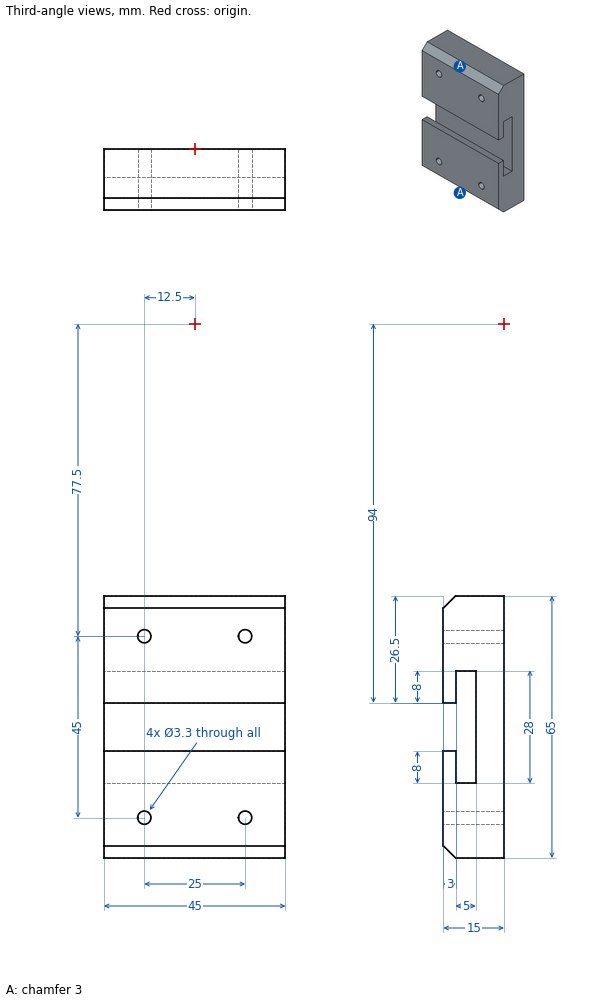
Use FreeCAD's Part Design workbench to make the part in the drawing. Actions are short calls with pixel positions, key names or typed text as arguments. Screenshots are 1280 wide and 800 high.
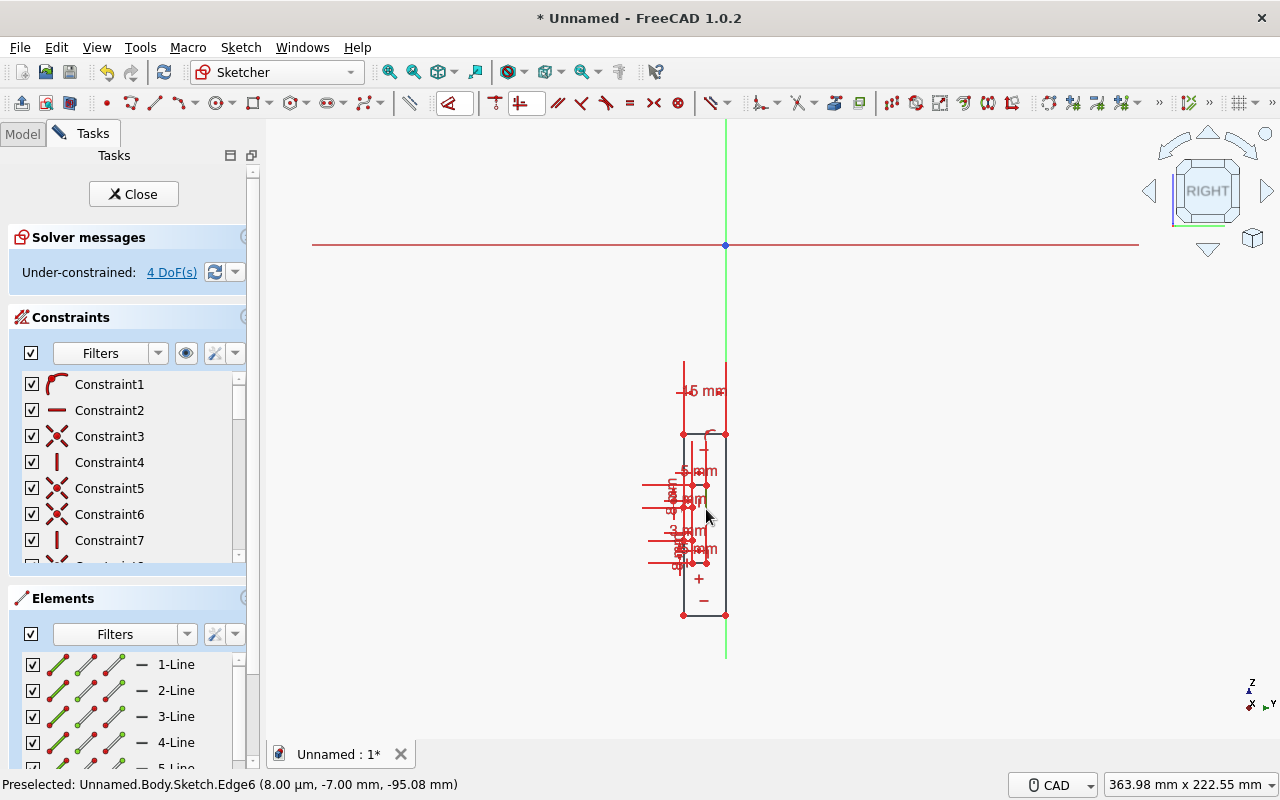
click(468, 104)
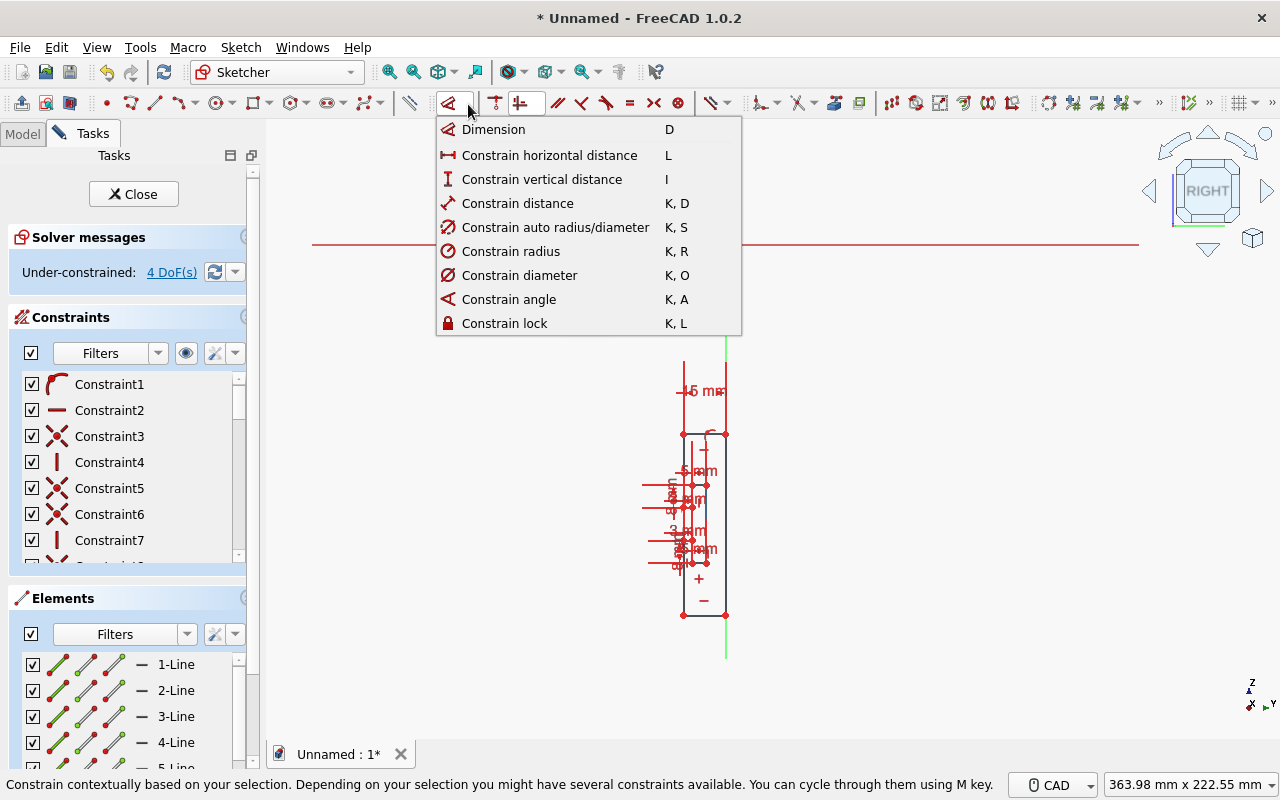
click(589, 179)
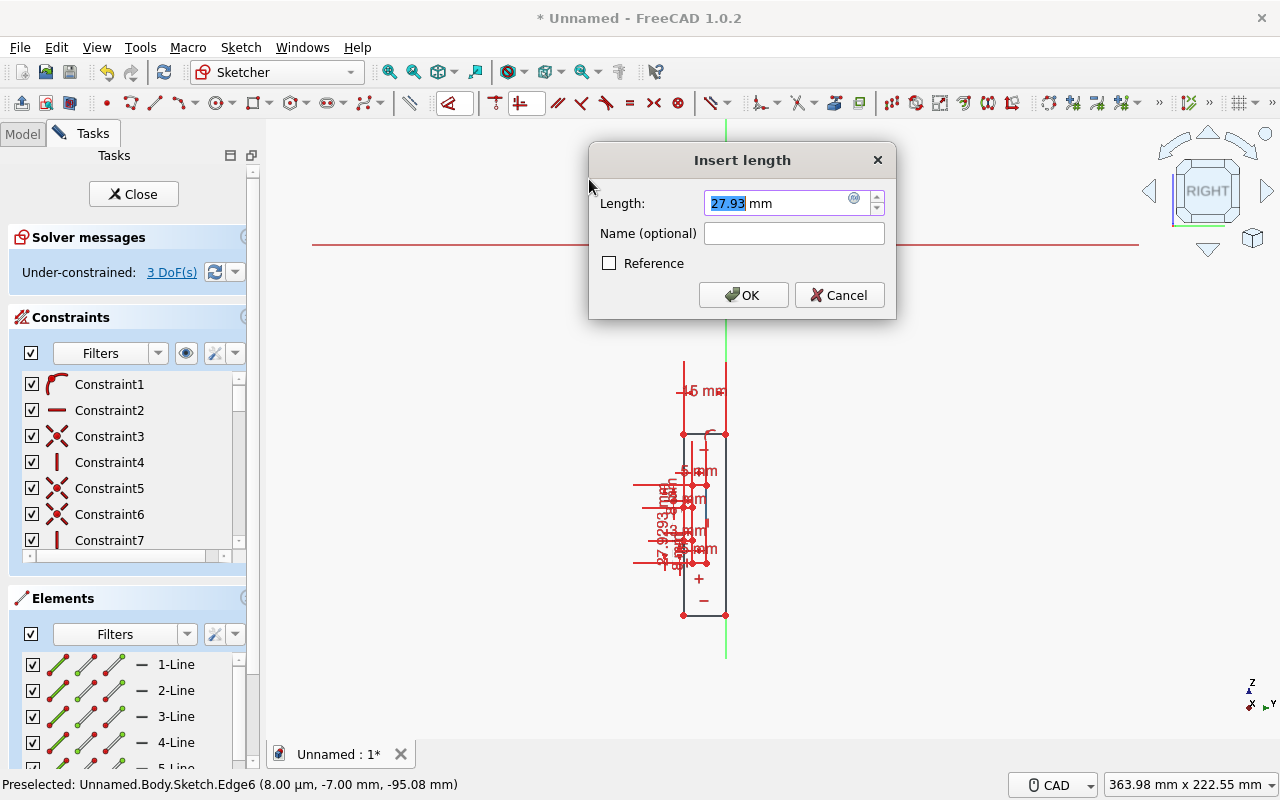
text(28)
key(Return)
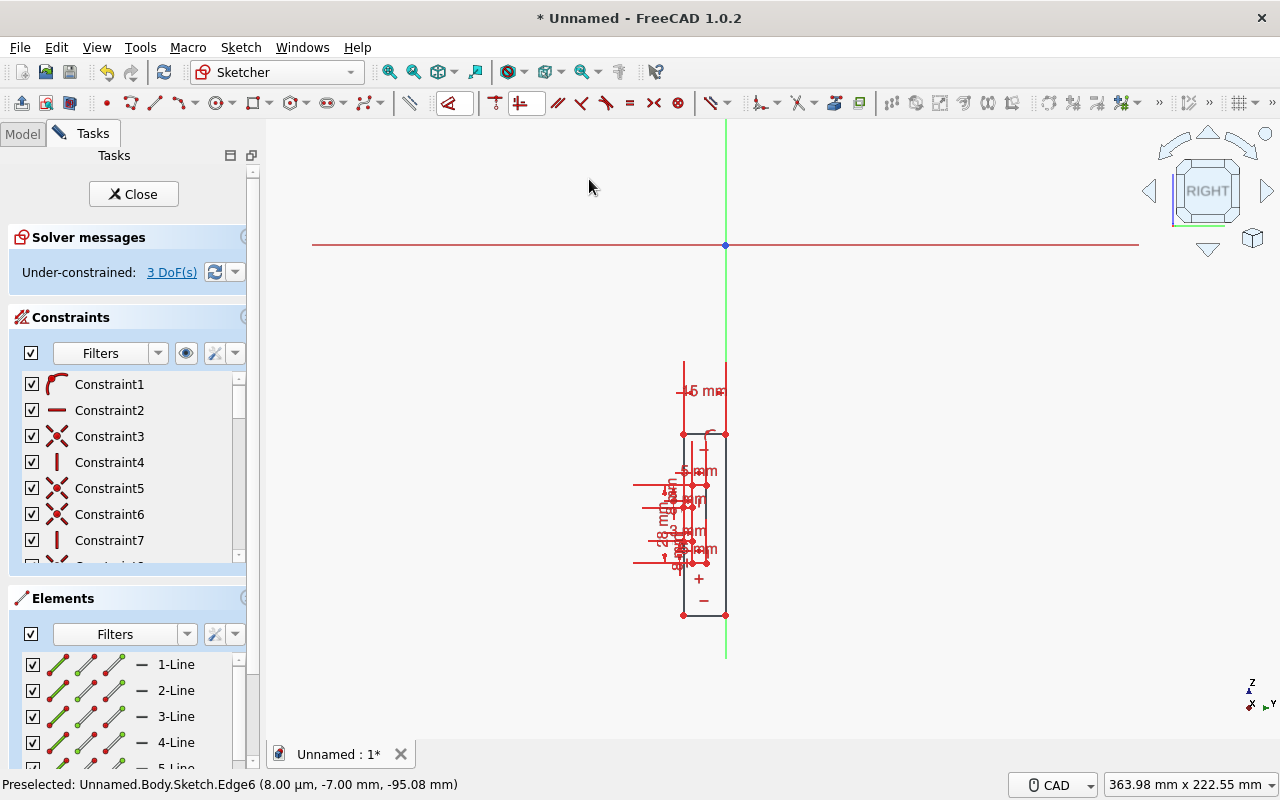
click(726, 561)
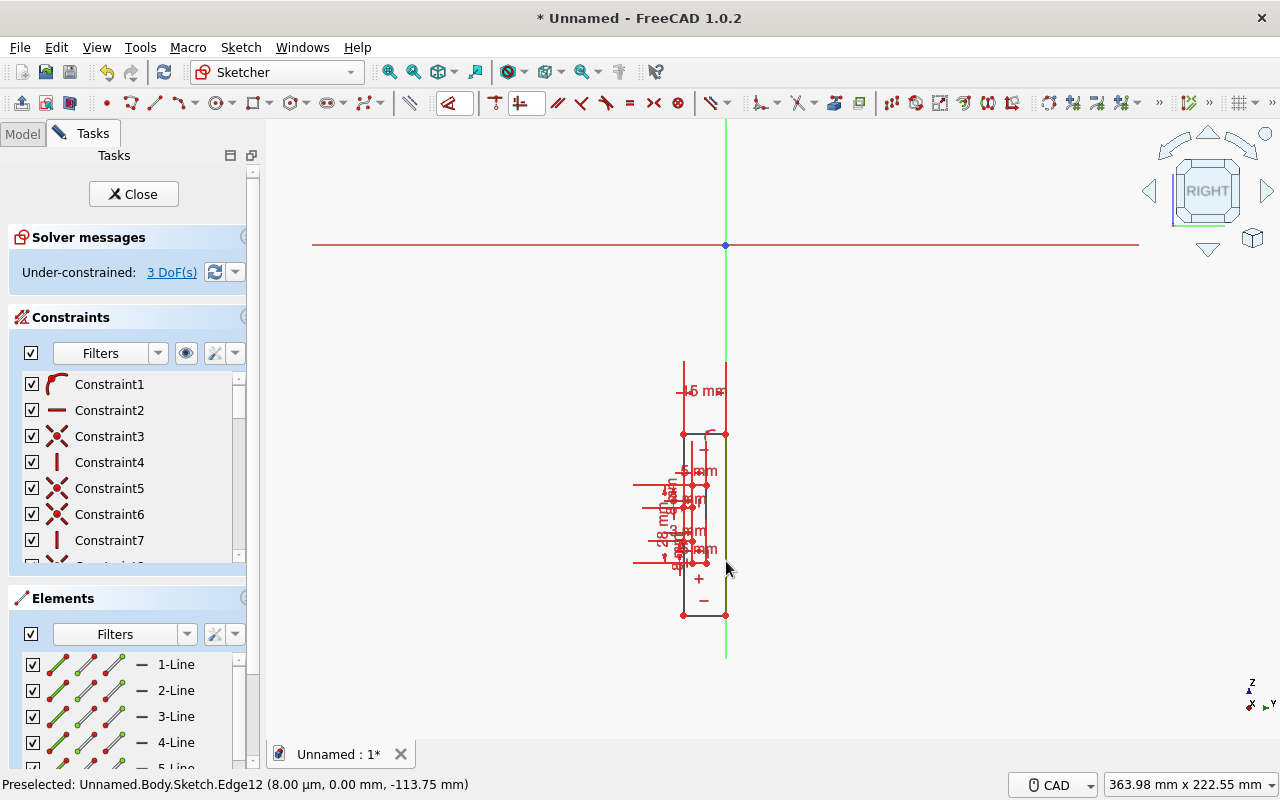
click(468, 104)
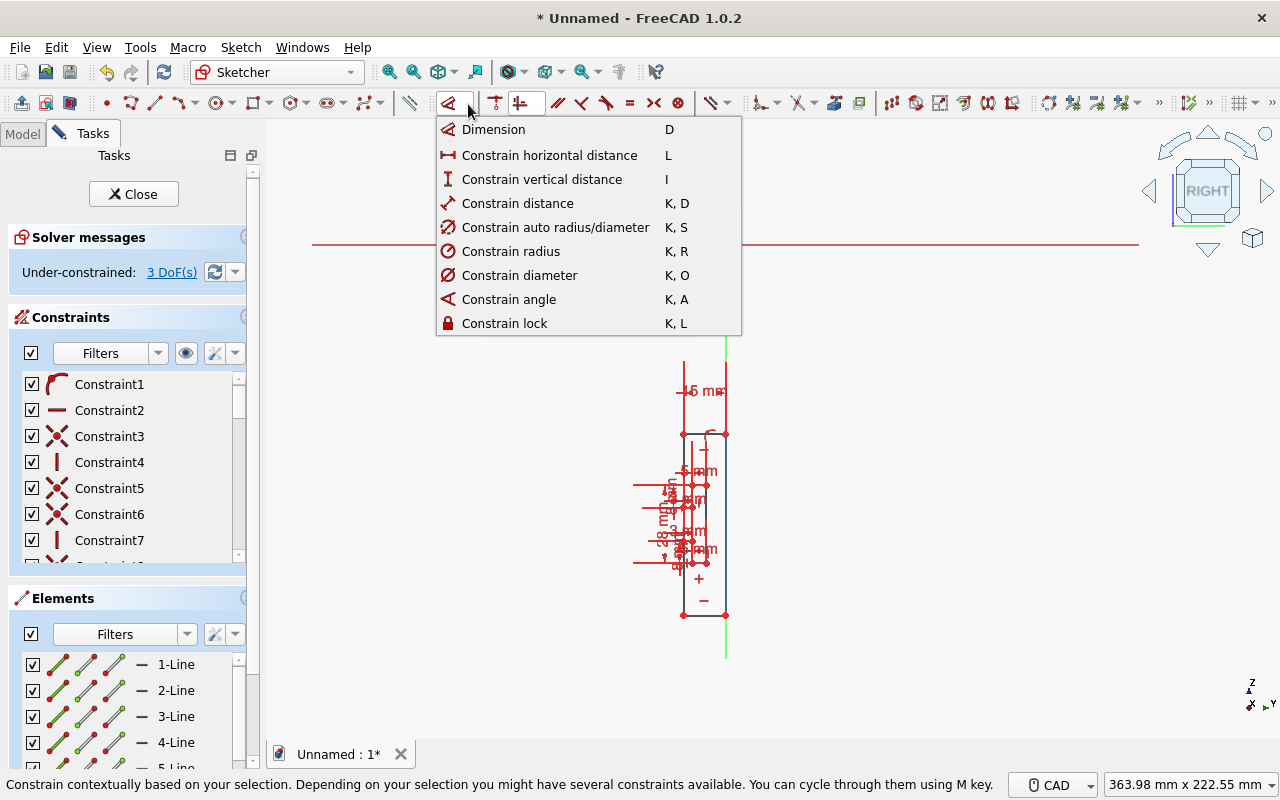
click(589, 179)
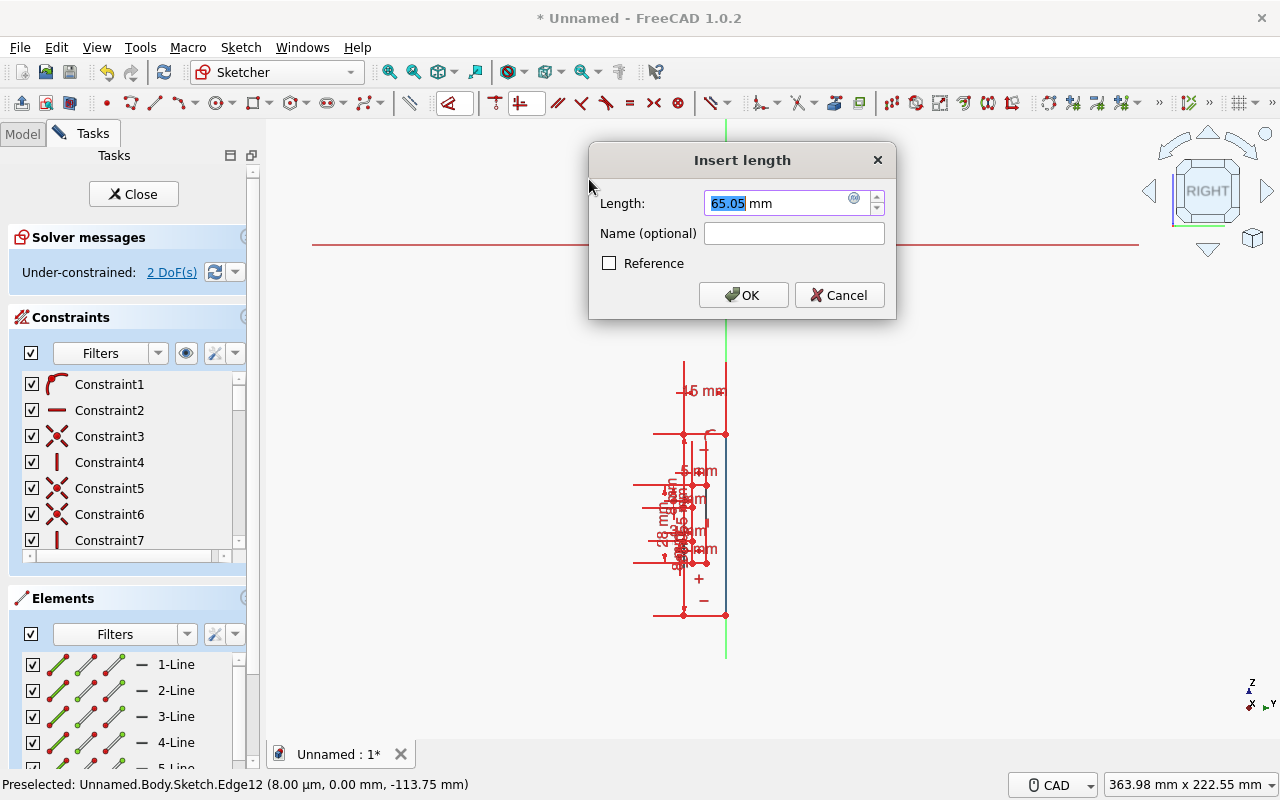
text(65)
key(Return)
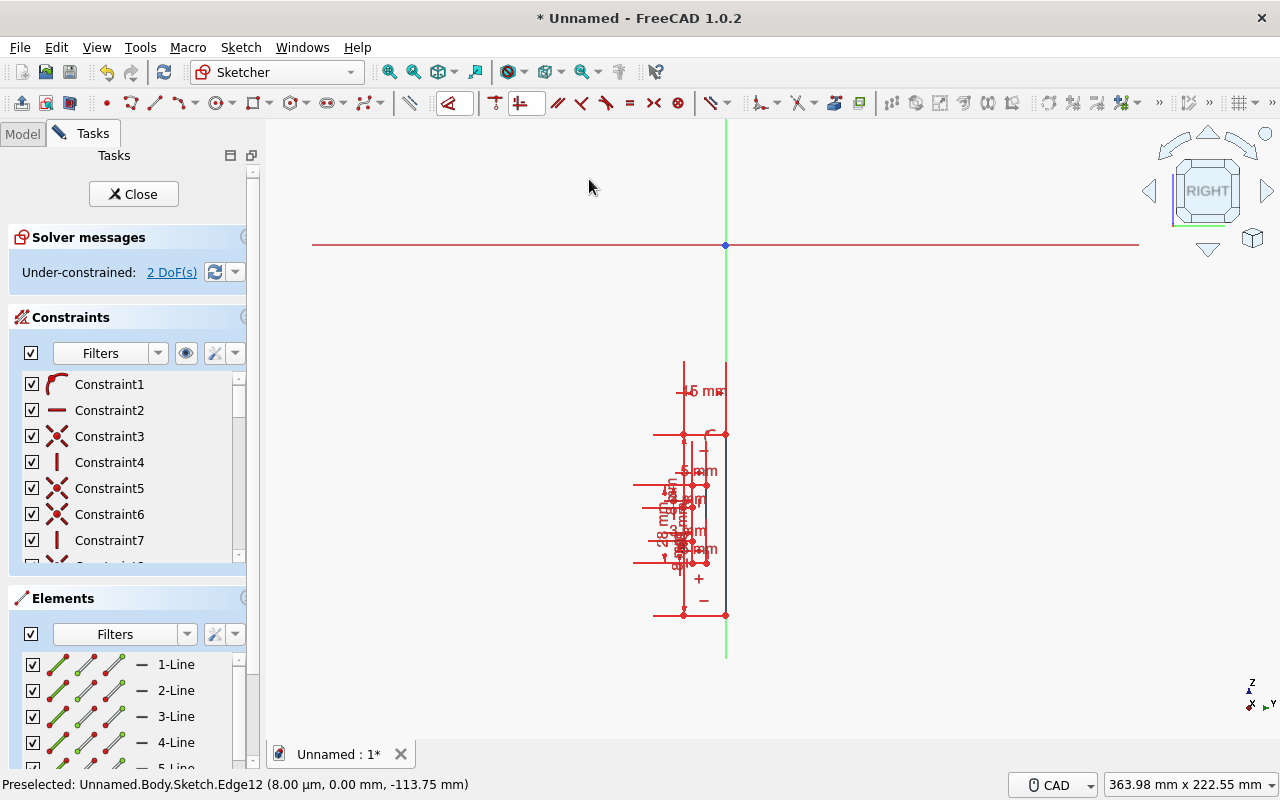
scroll(684, 508, up, 2)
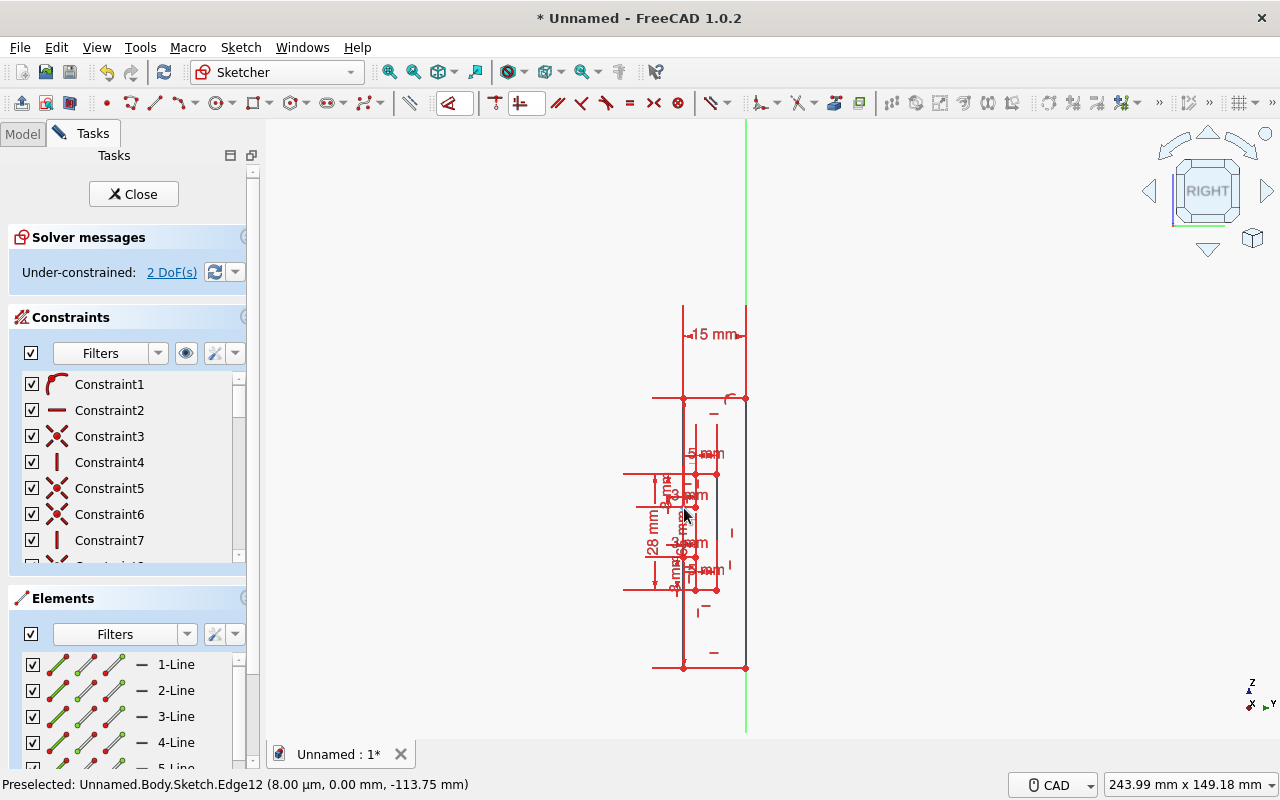
click(683, 507)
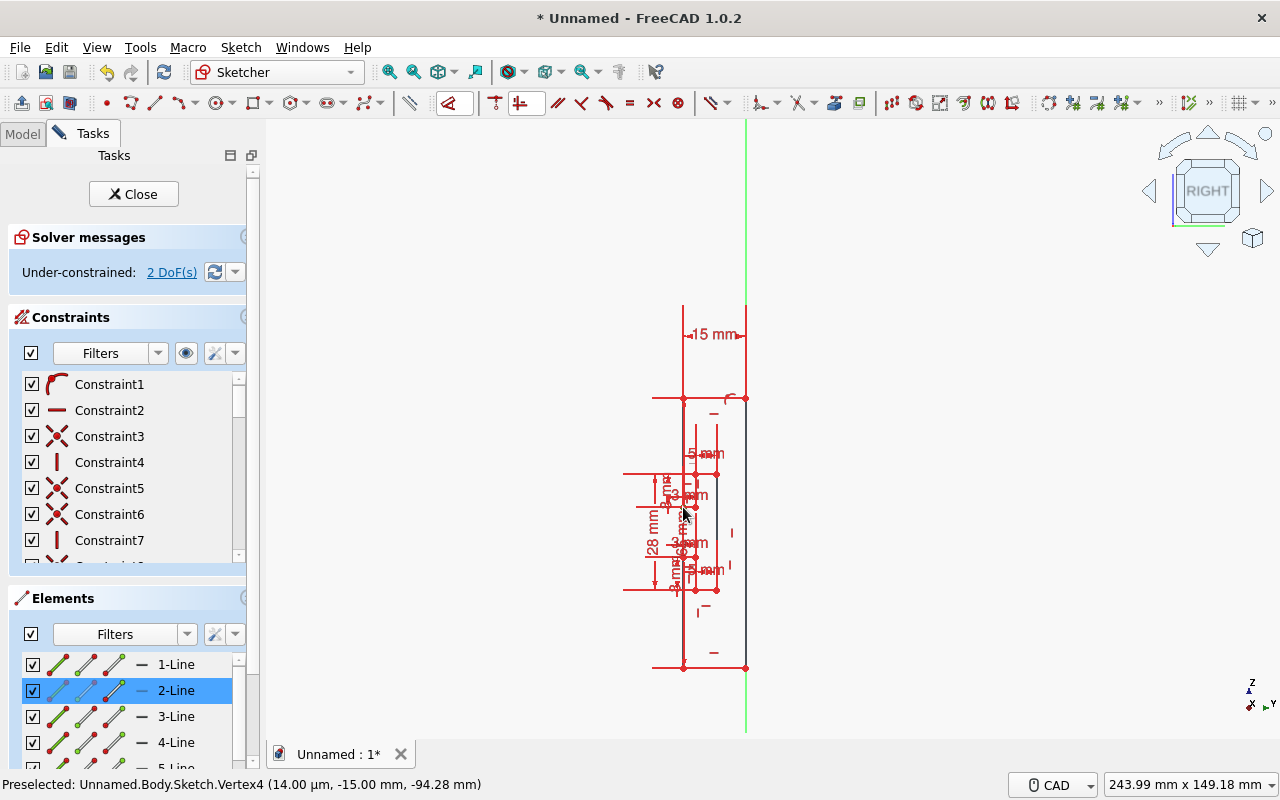
key(i)